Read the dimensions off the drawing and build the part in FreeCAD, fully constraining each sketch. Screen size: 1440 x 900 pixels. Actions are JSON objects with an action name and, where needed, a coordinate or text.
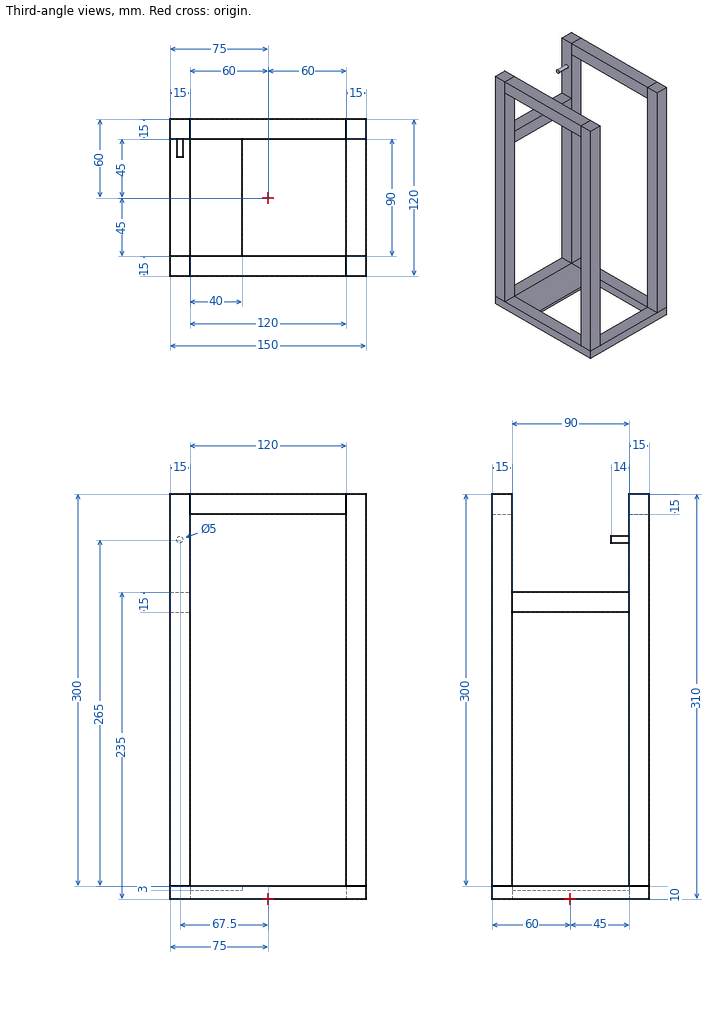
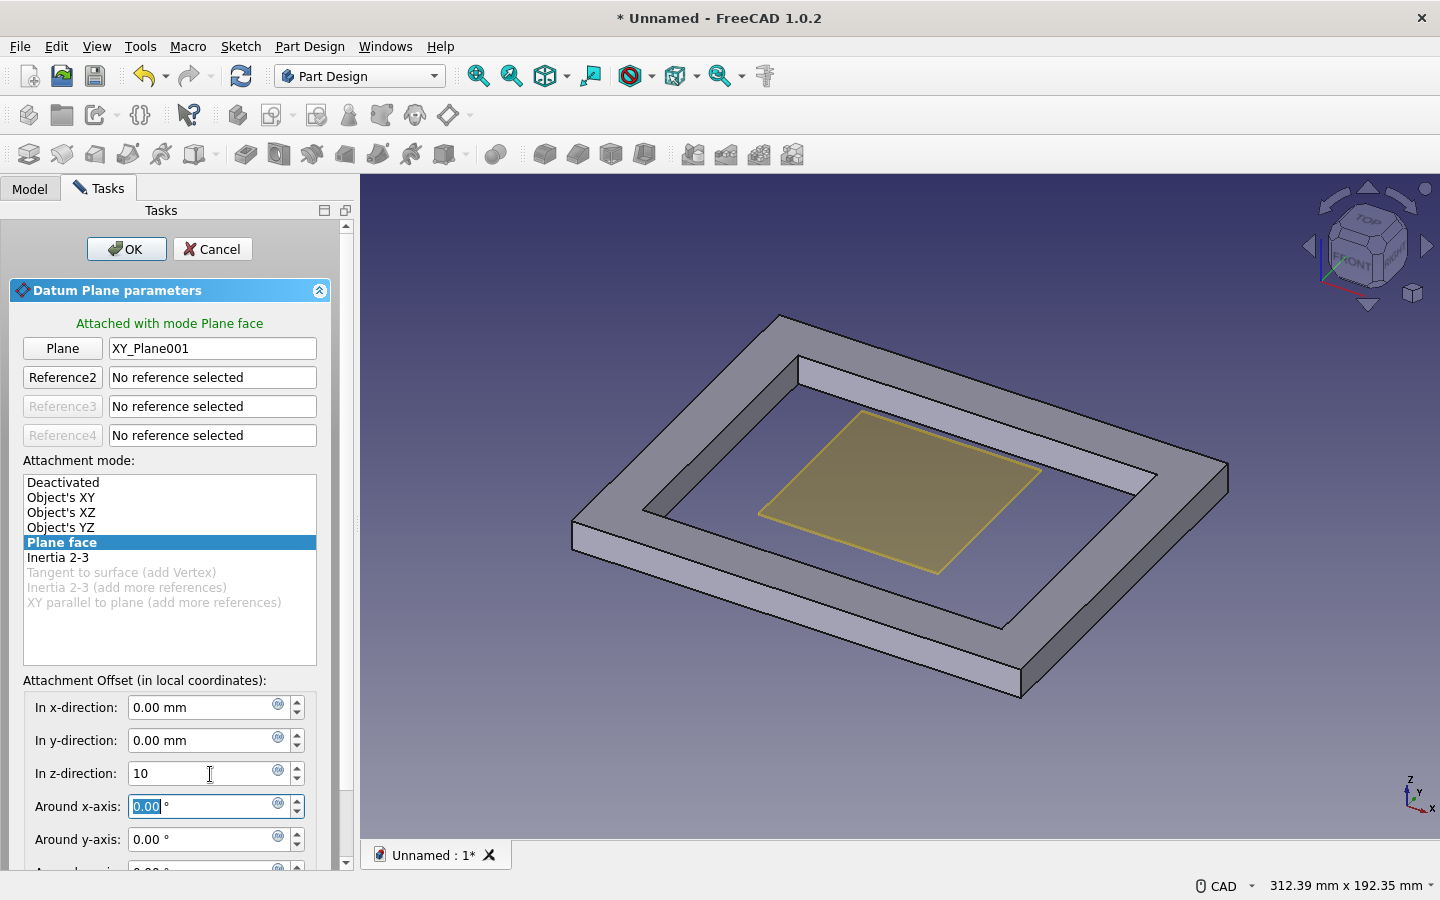
{"action": "left_click", "coordinate": [127, 249]}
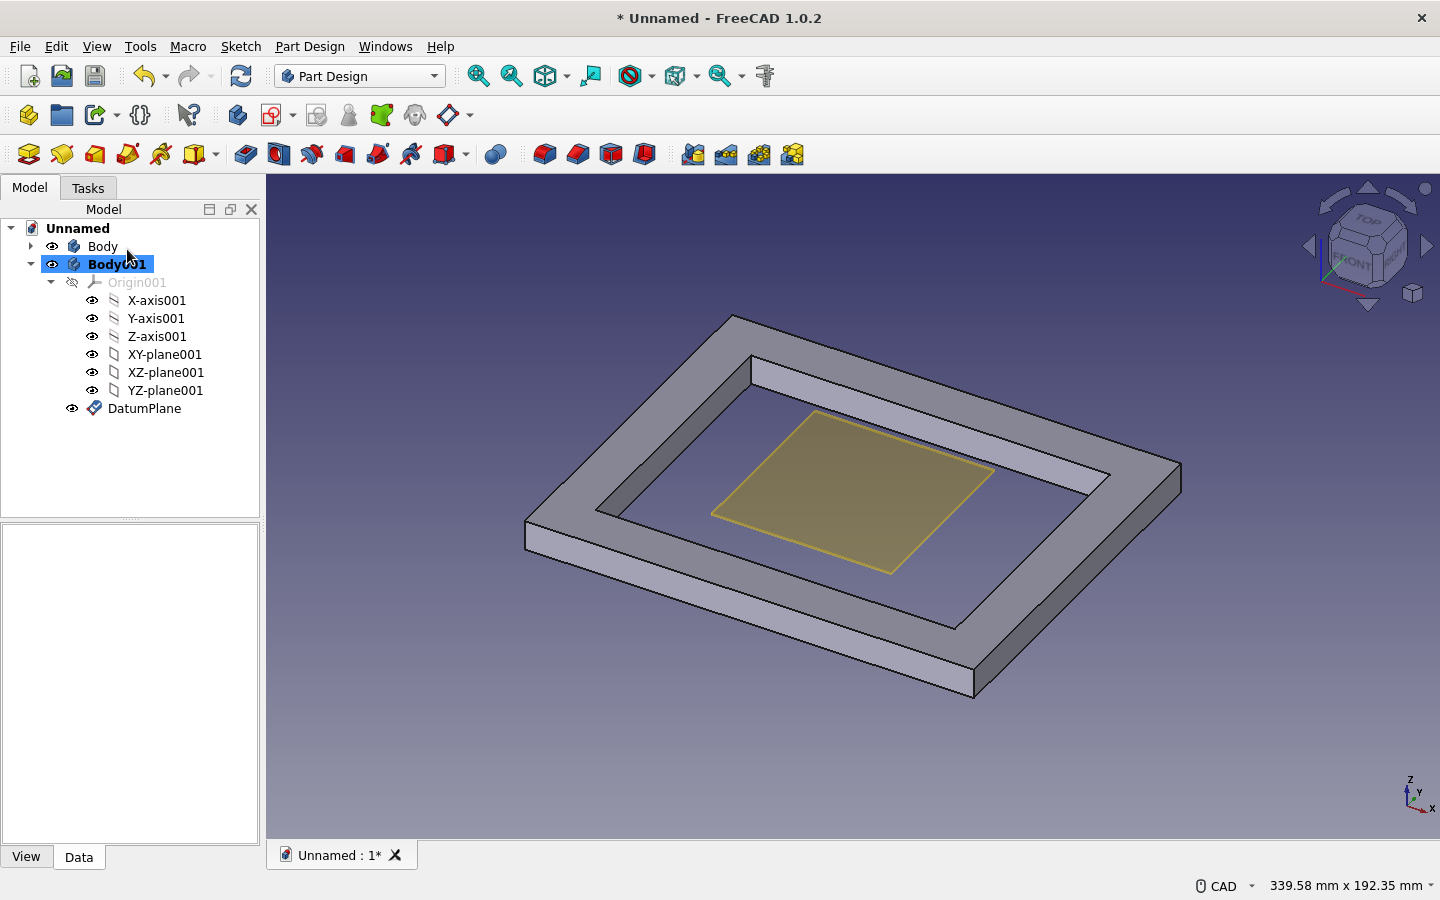
{"action": "left_click", "coordinate": [117, 408]}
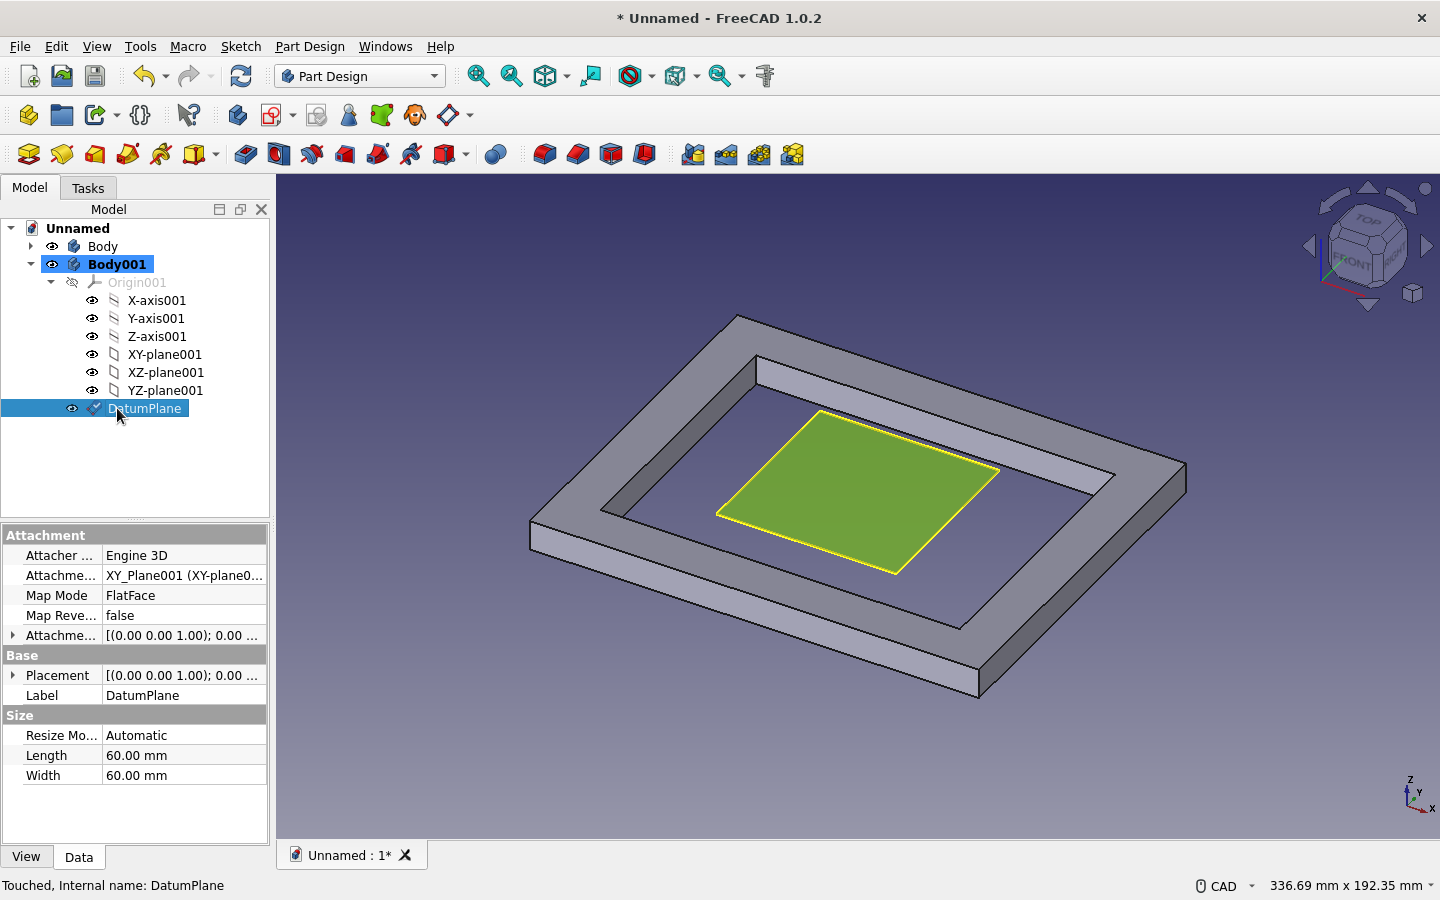
{"action": "left_click", "coordinate": [270, 116]}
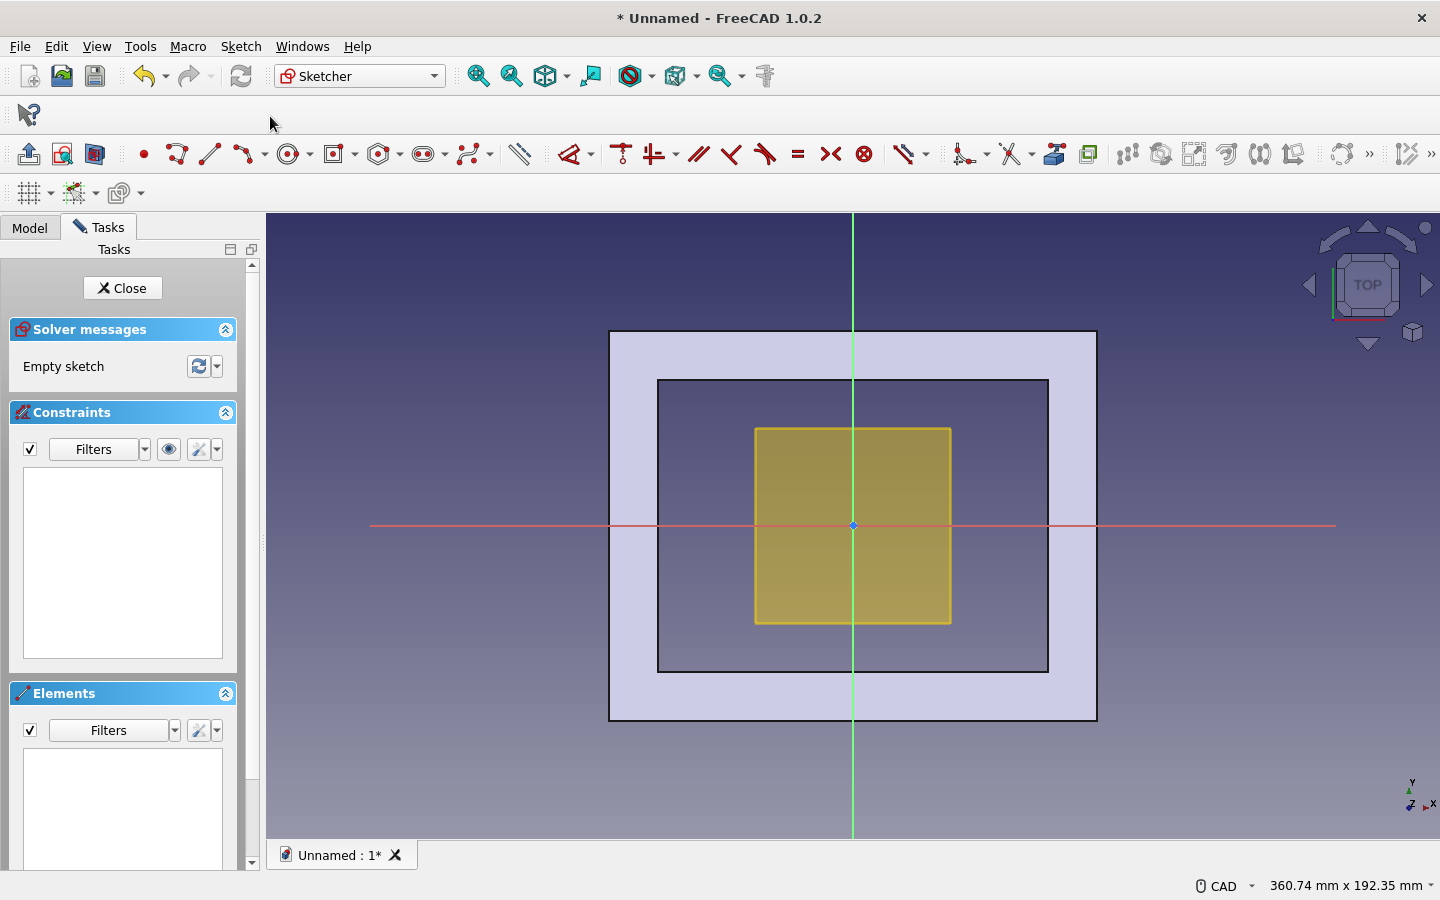
{"action": "scroll", "coordinate": [614, 334], "scroll_direction": "up", "scroll_amount": 11}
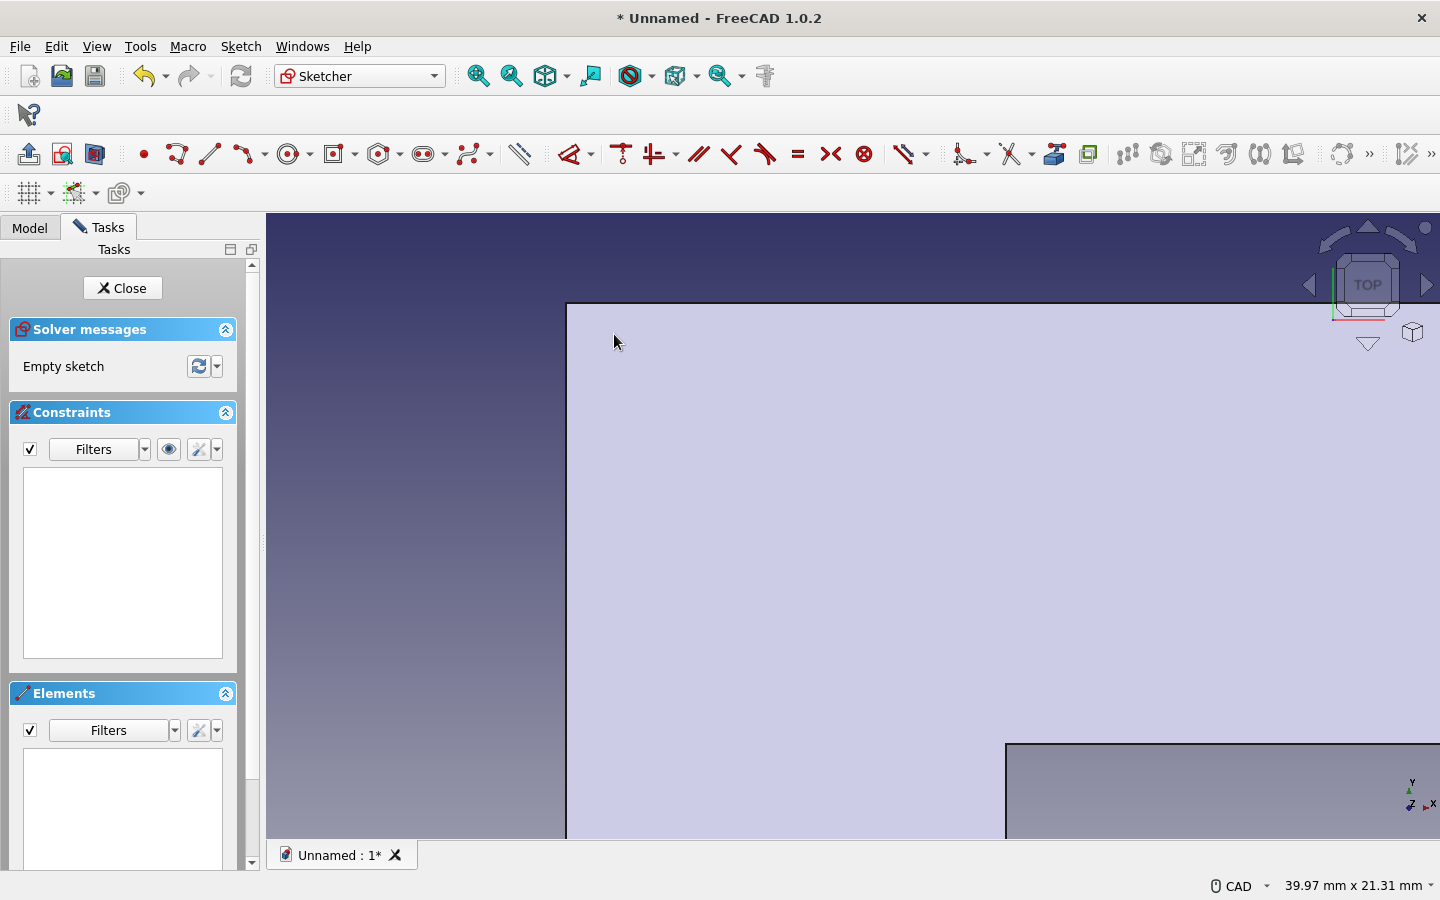
{"action": "left_click", "coordinate": [354, 154]}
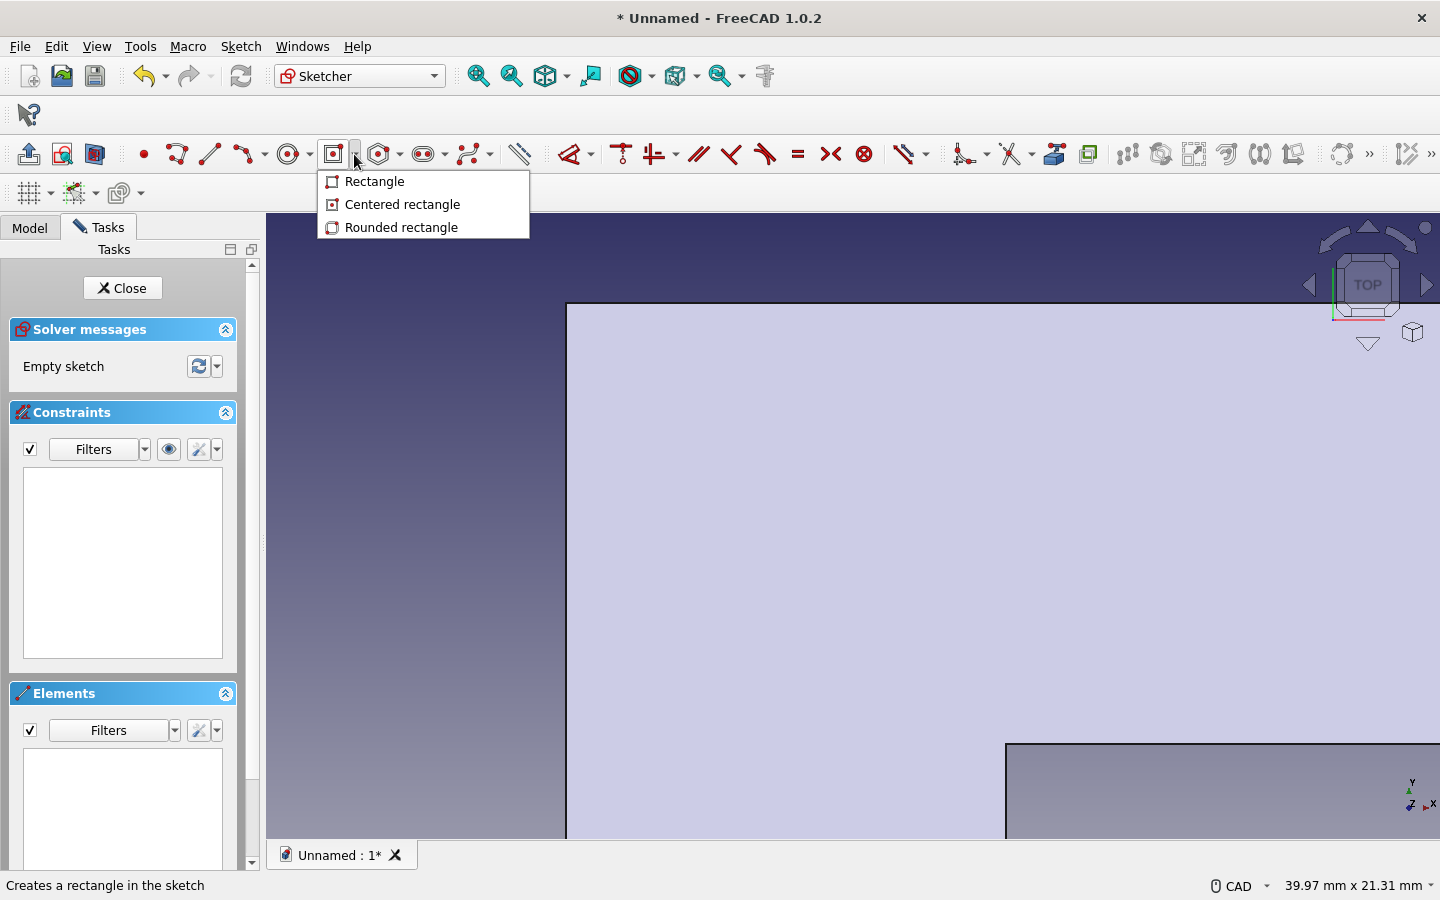
{"action": "left_click", "coordinate": [424, 182]}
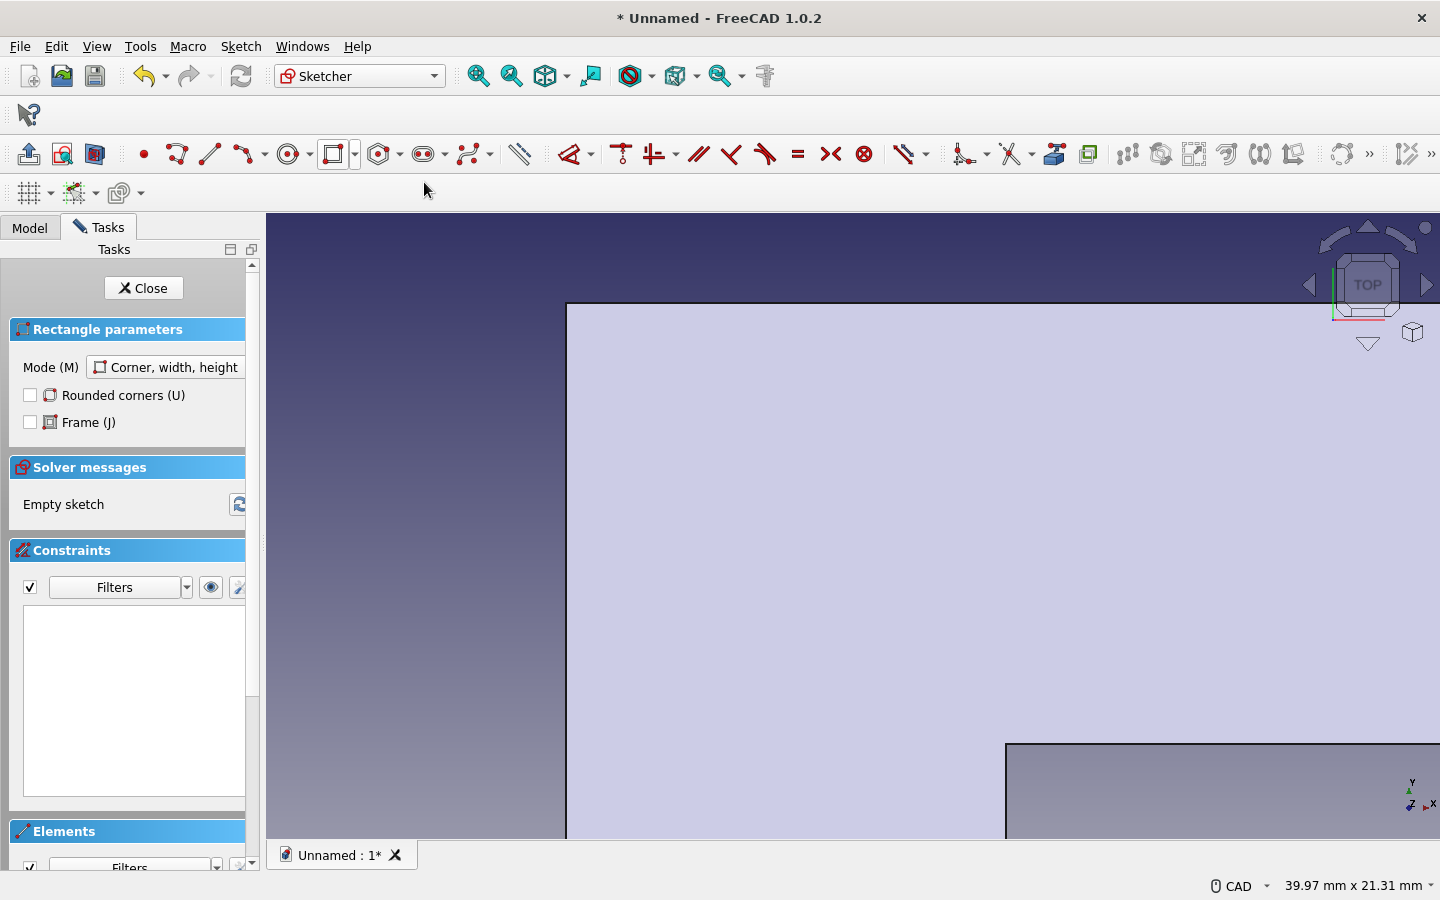
{"action": "left_click", "coordinate": [566, 303]}
{"action": "left_click", "coordinate": [1006, 744]}
{"action": "key", "text": "Escape"}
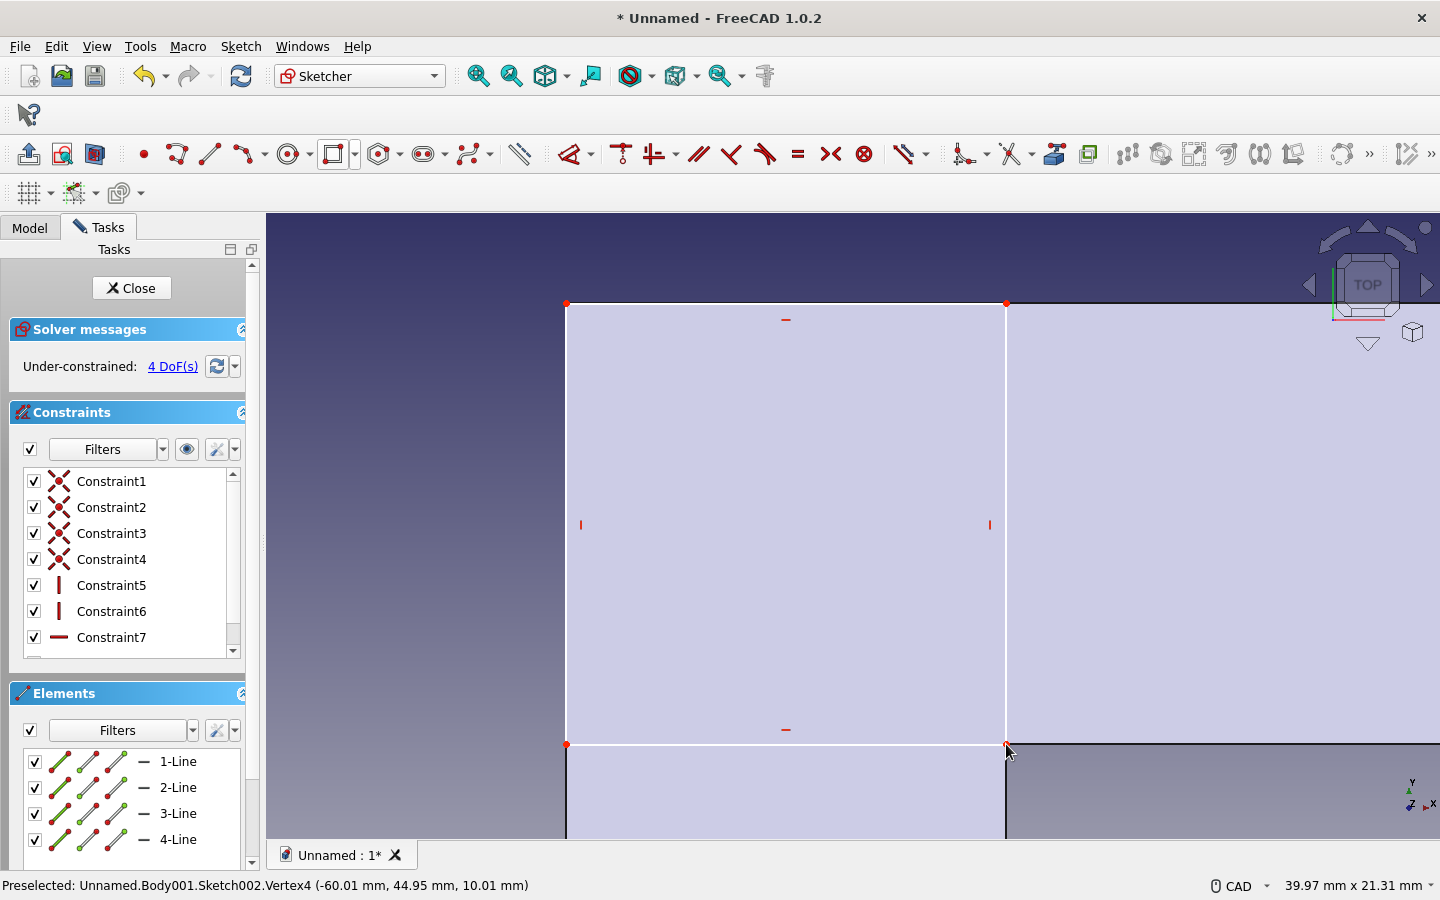
{"action": "left_click", "coordinate": [568, 154]}